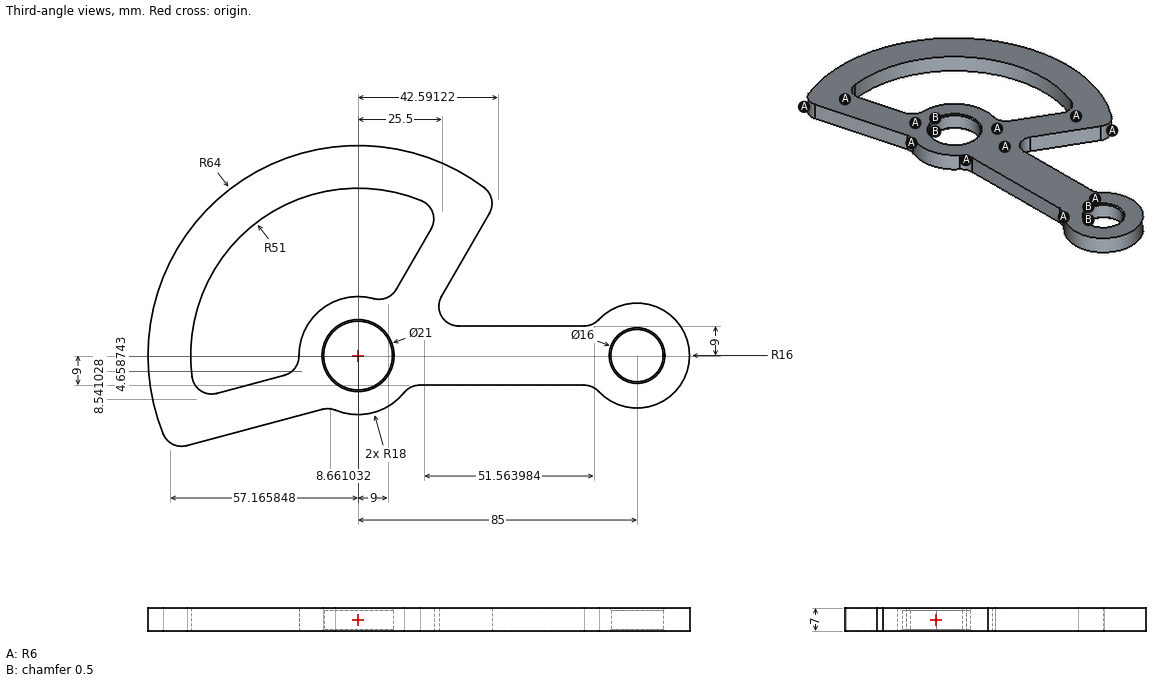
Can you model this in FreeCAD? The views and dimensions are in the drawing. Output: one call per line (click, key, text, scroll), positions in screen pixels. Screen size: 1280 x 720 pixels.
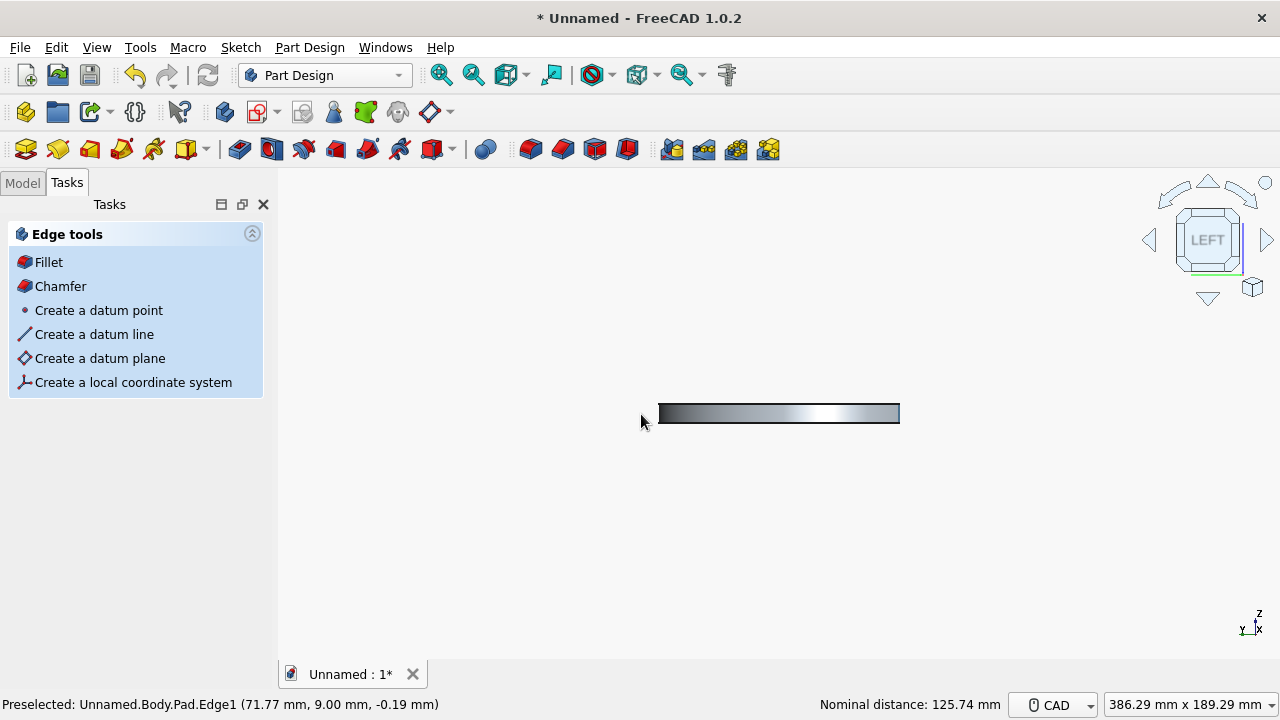
click(442, 76)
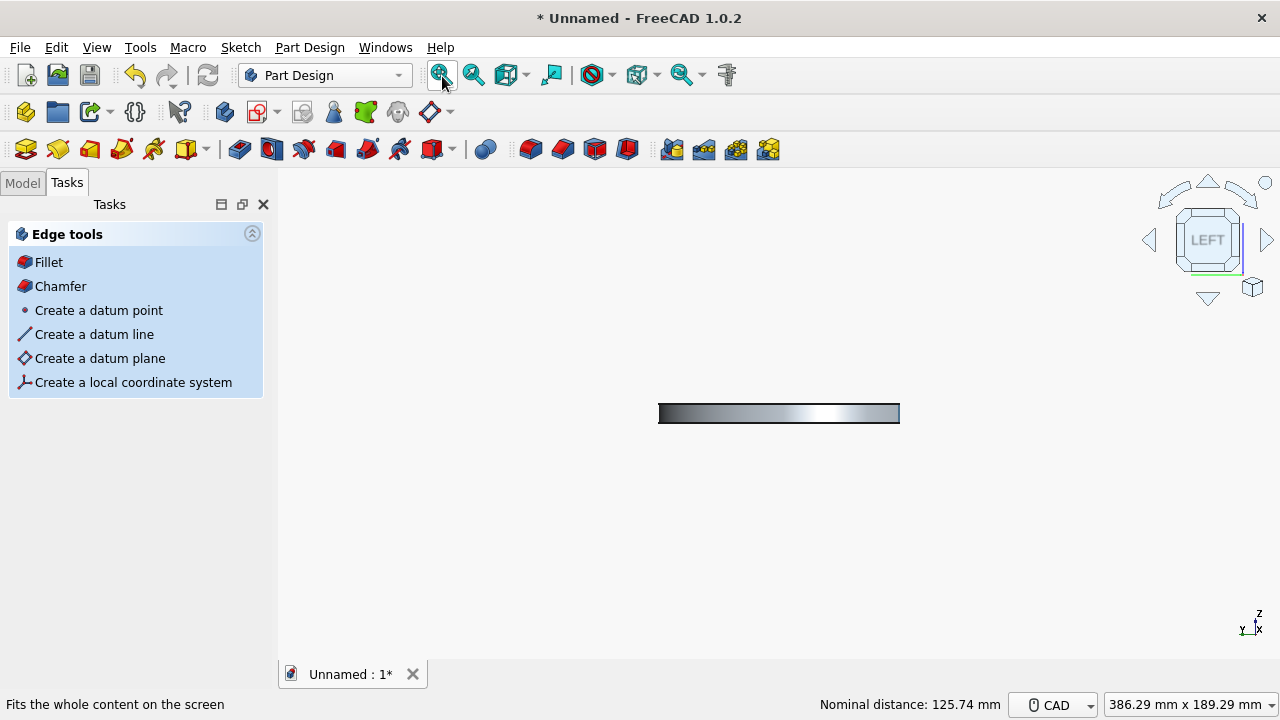
scroll(848, 412, up, 4)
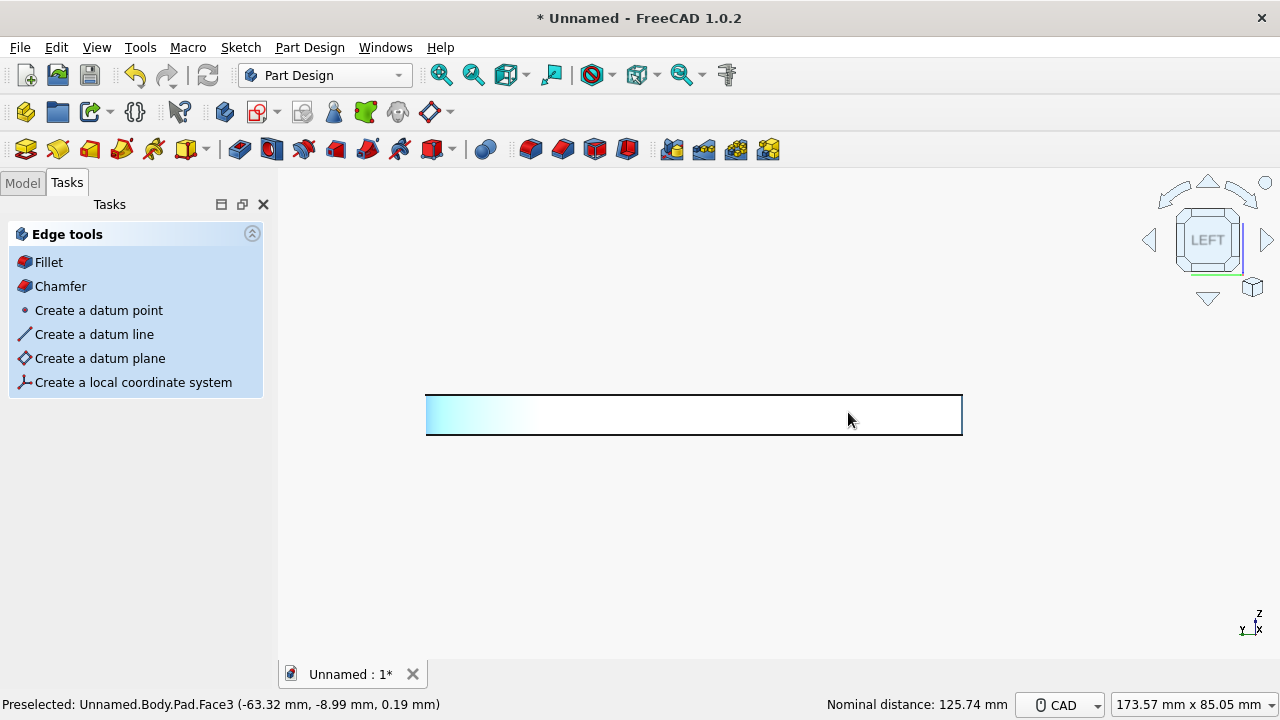
key(v)
key(f)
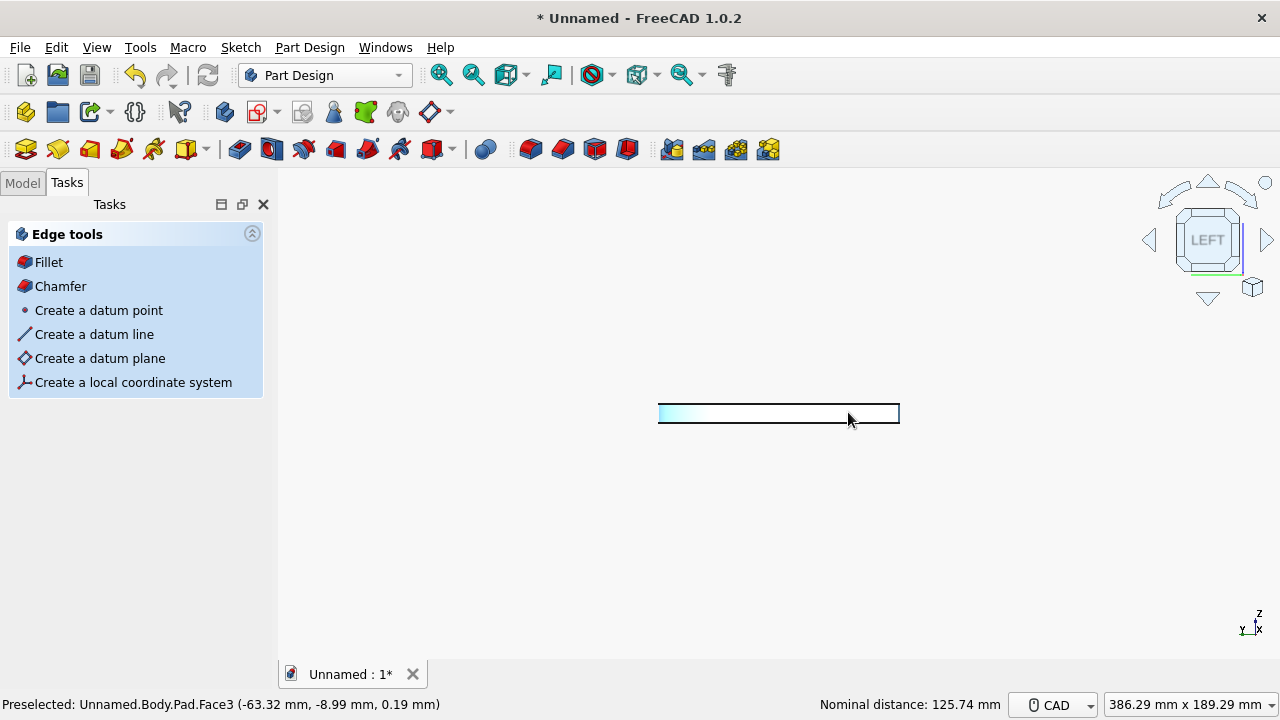
key(v)
key(3)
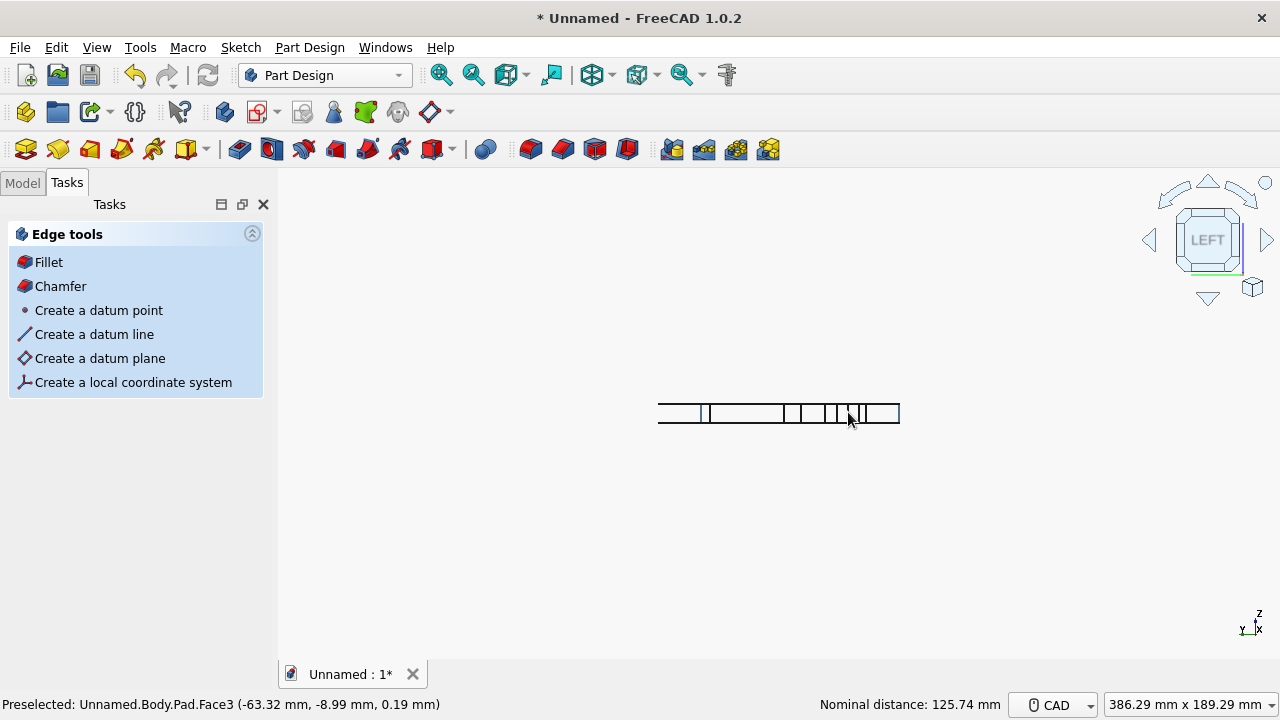
key(0)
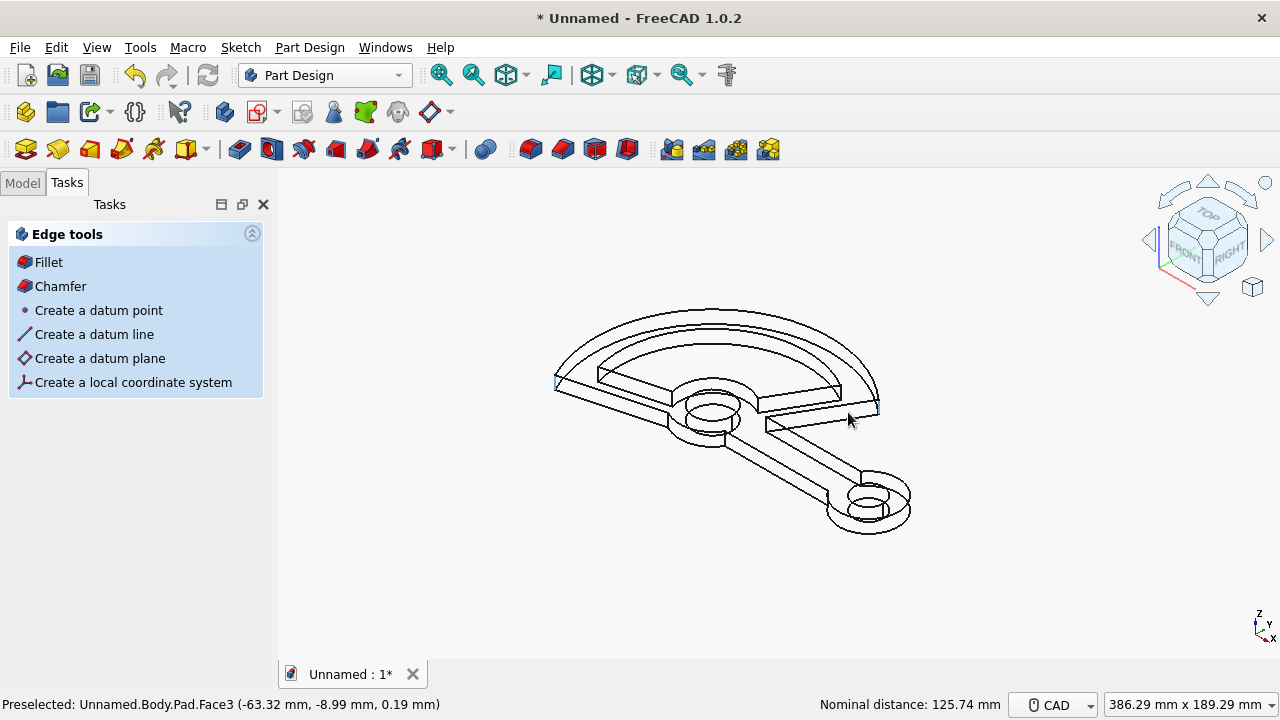
click(725, 438, ctrl)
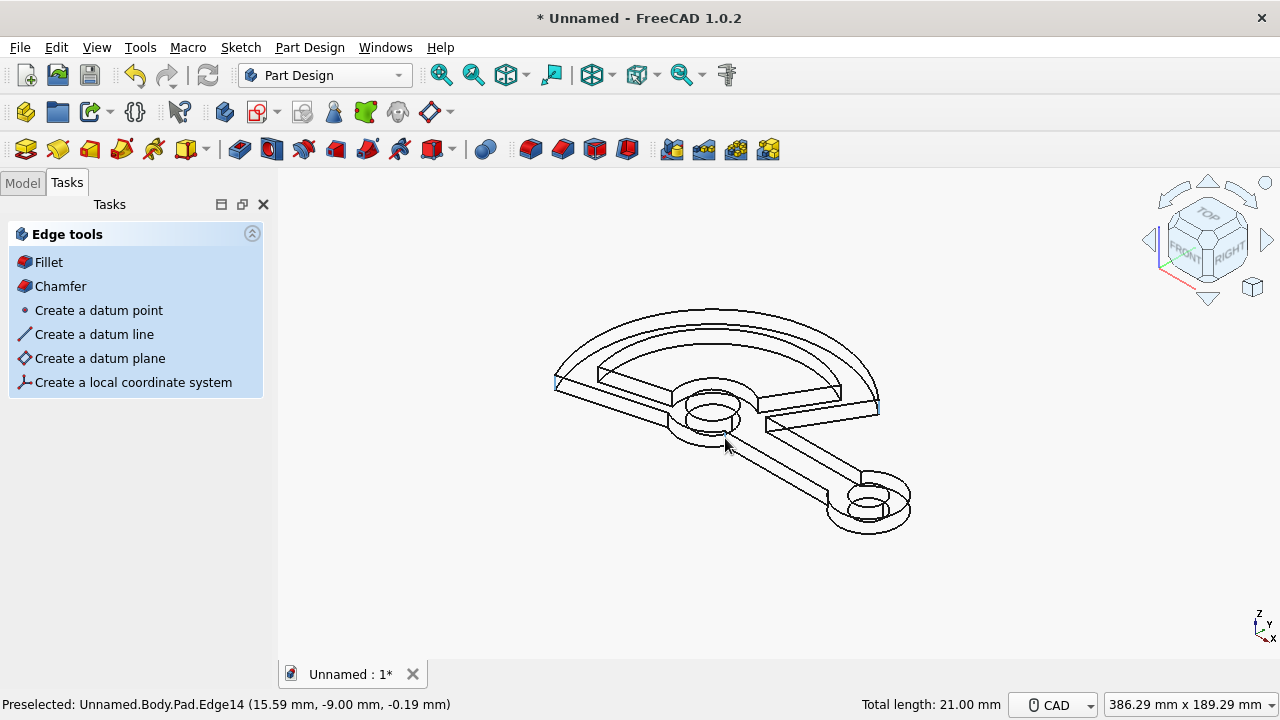
click(668, 424, ctrl)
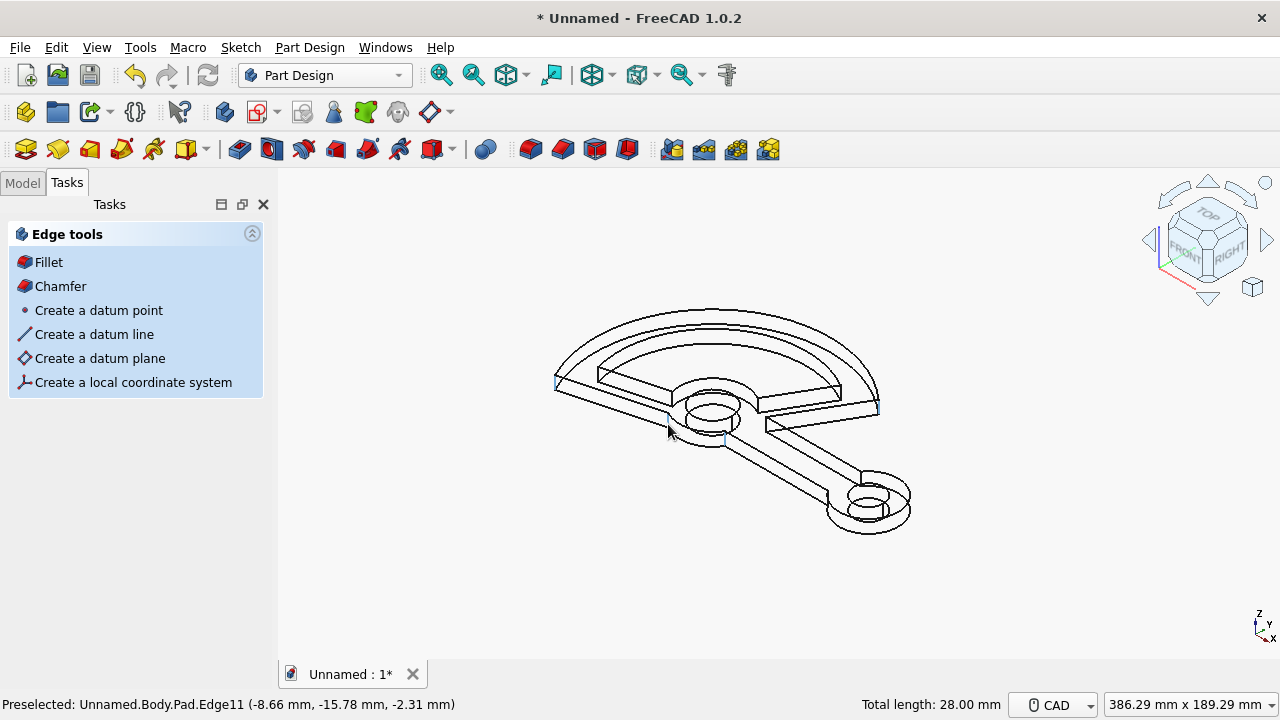
click(766, 425, ctrl)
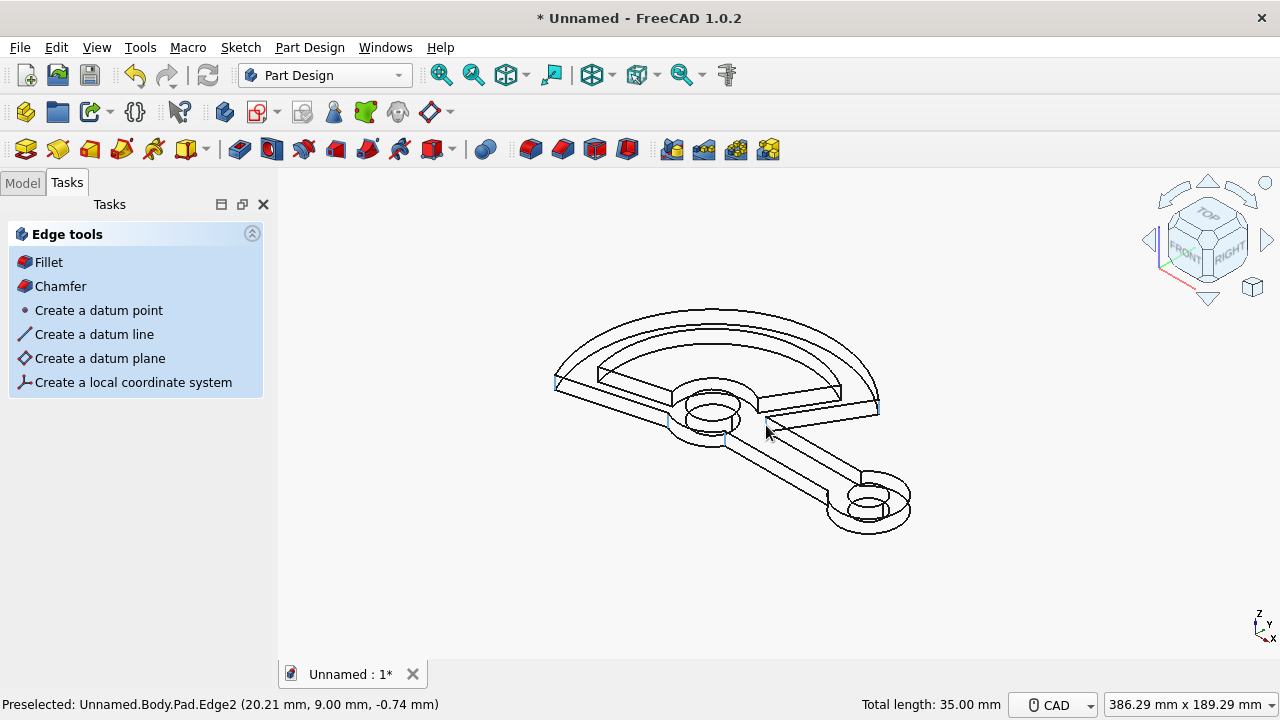
click(672, 398, ctrl)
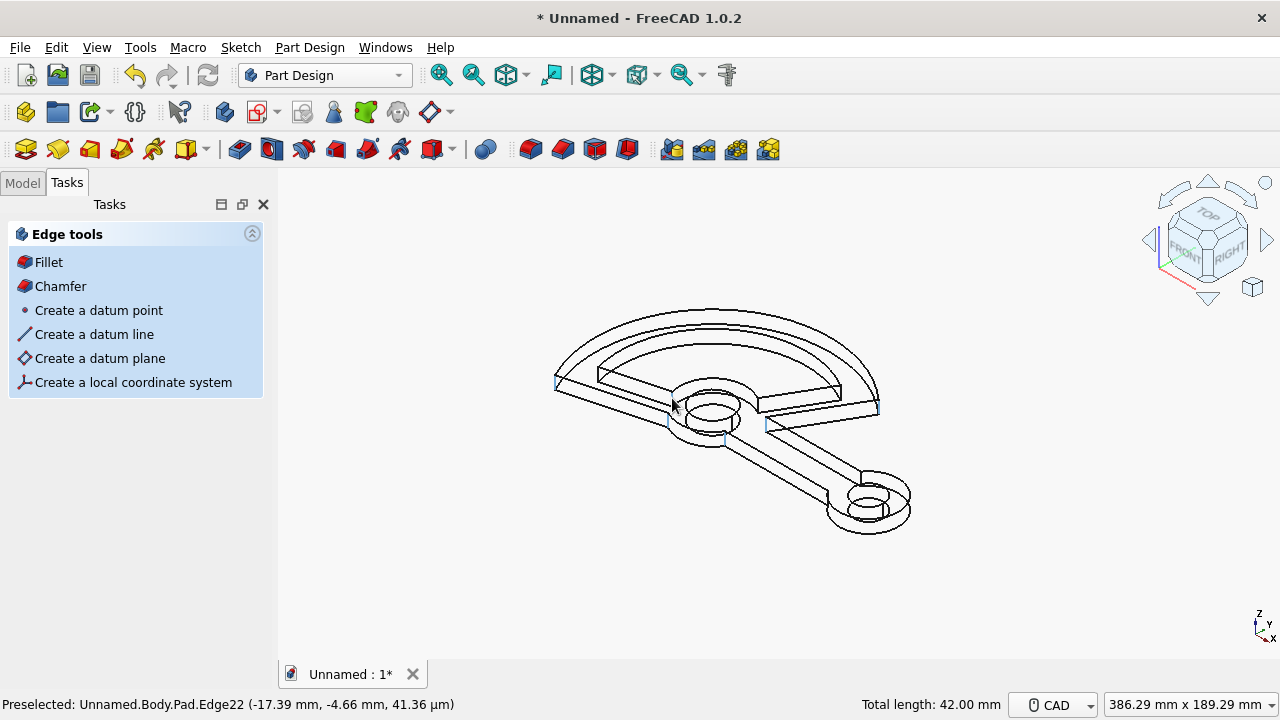
click(758, 405, ctrl)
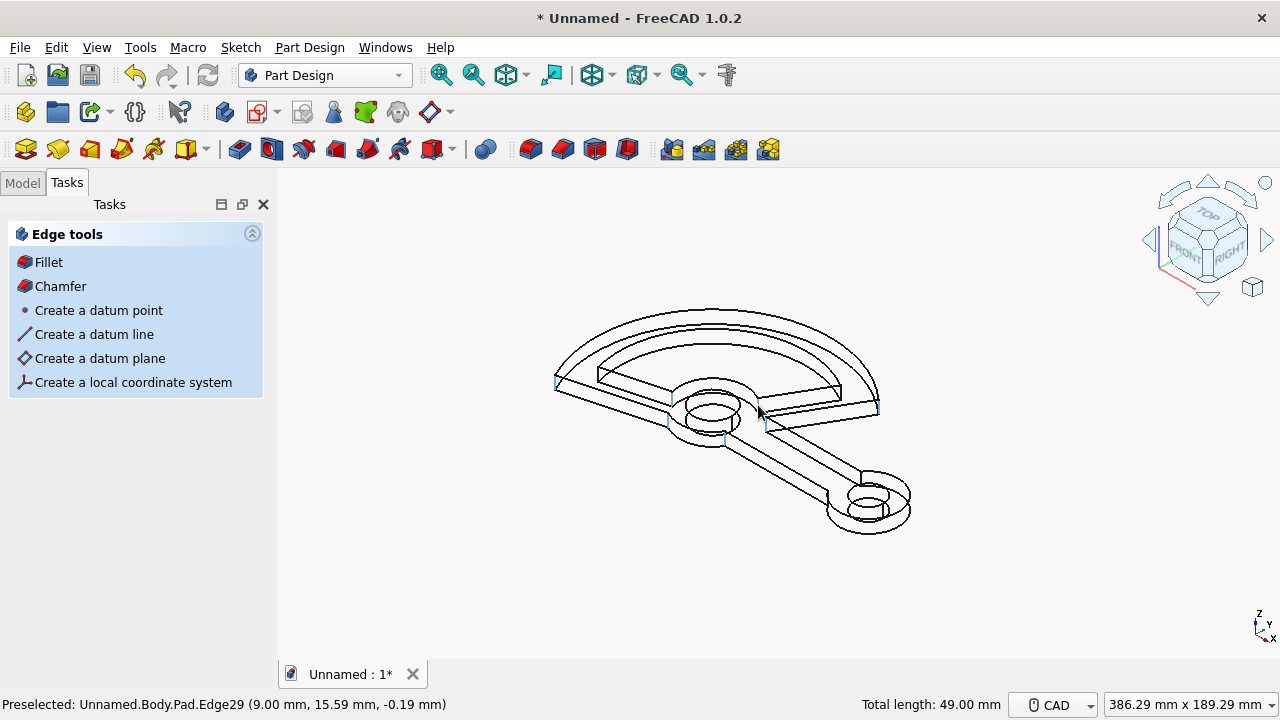
click(841, 392, ctrl)